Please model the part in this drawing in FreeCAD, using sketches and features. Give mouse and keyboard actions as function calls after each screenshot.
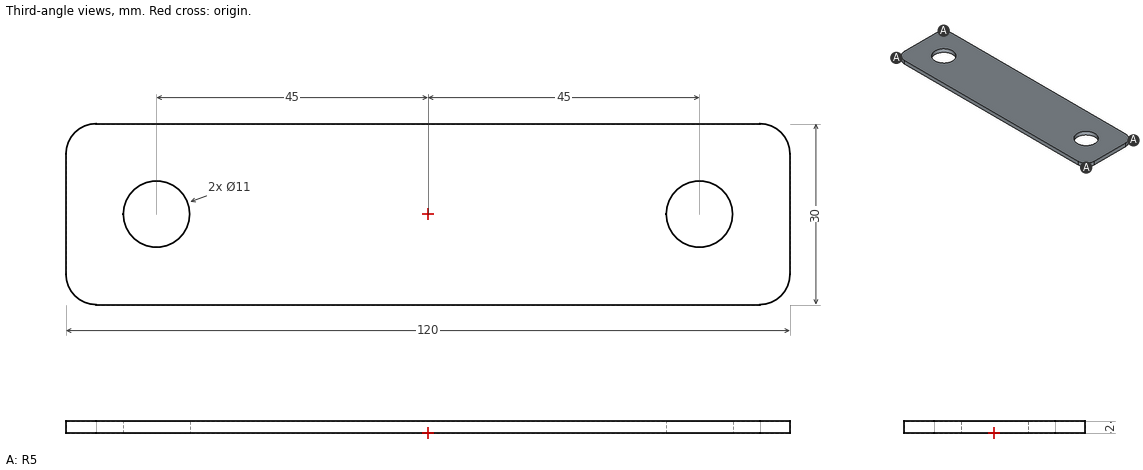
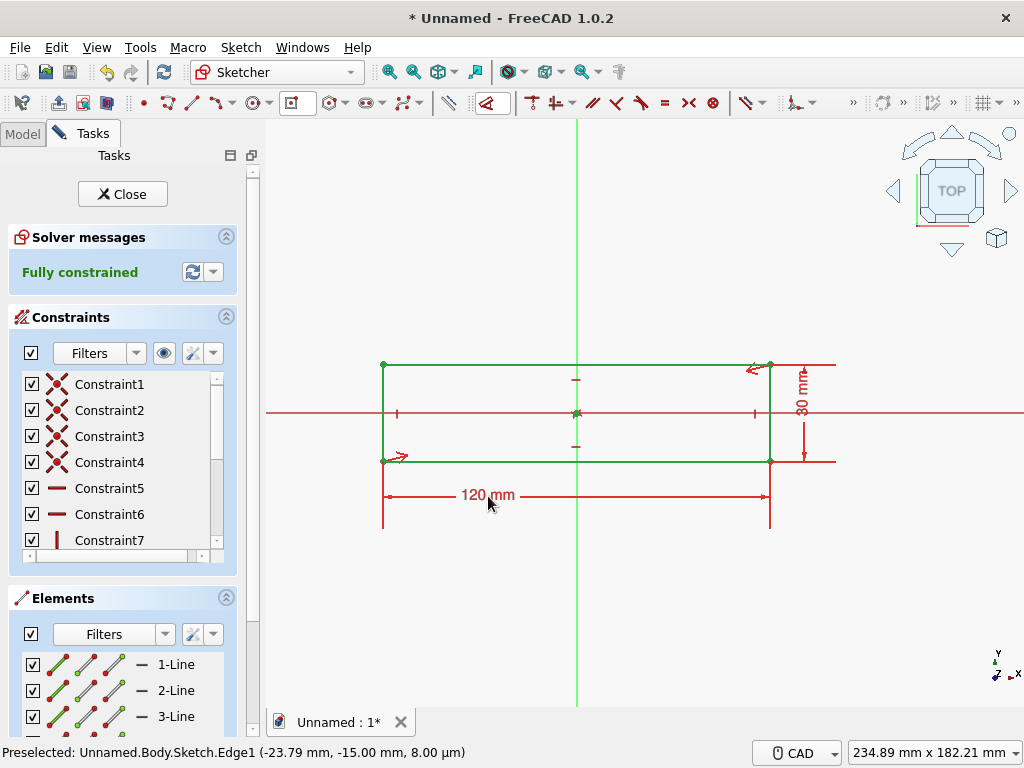
click(123, 194)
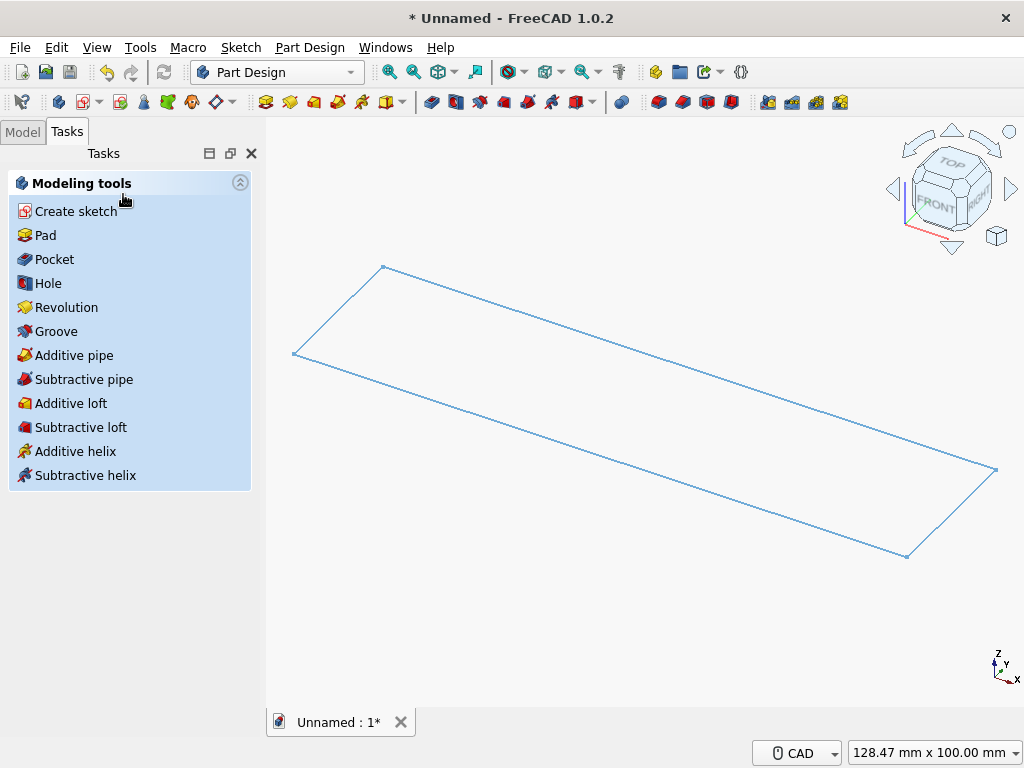
click(266, 102)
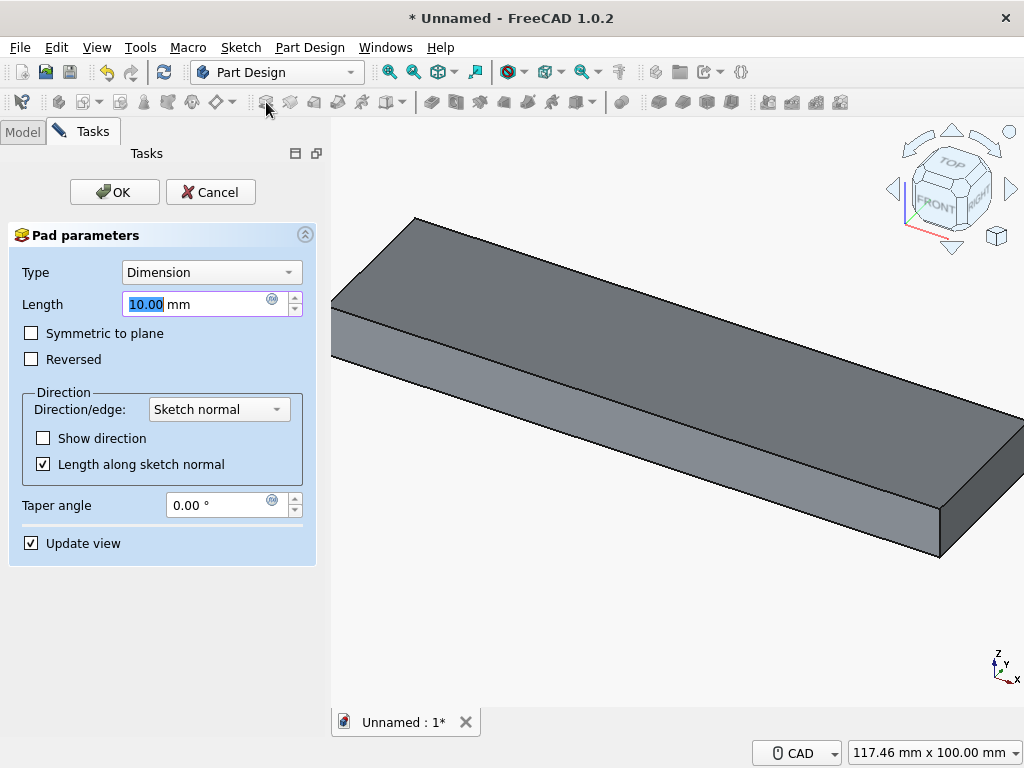
text(2)
key(Tab)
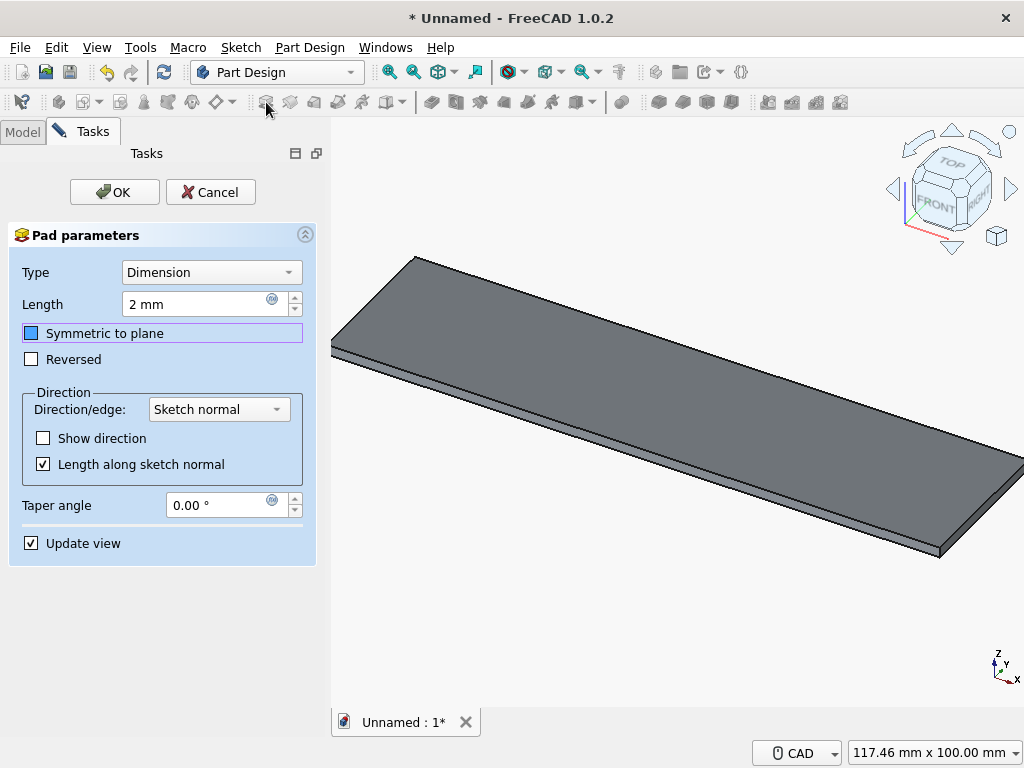
click(115, 192)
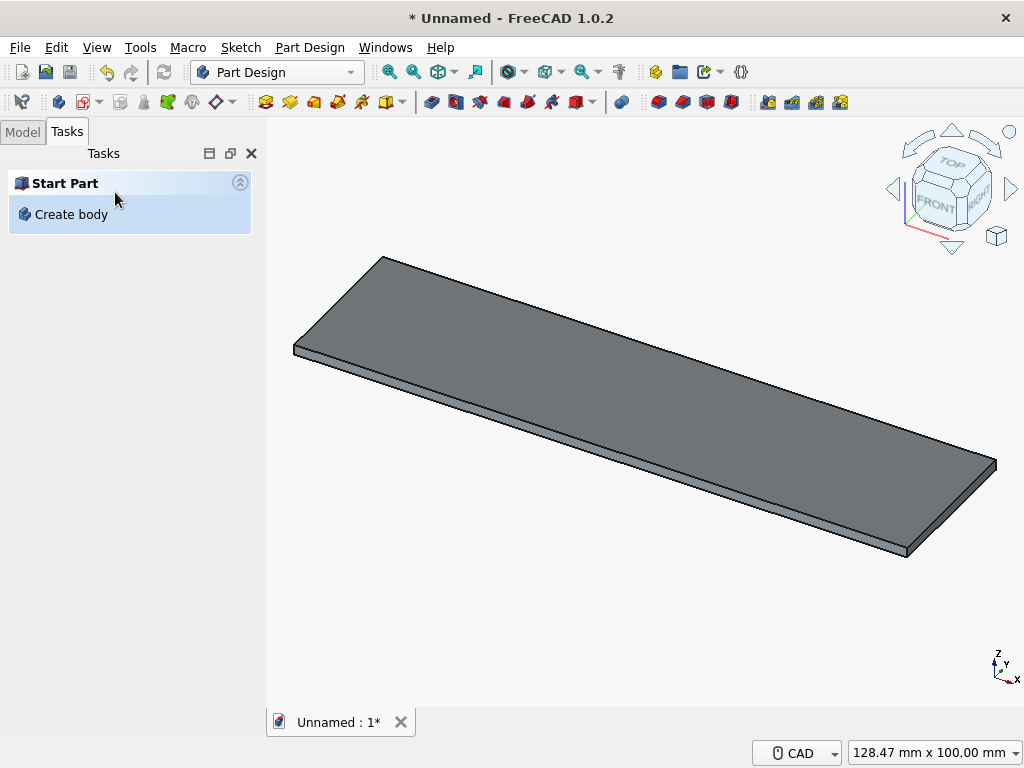
click(84, 102)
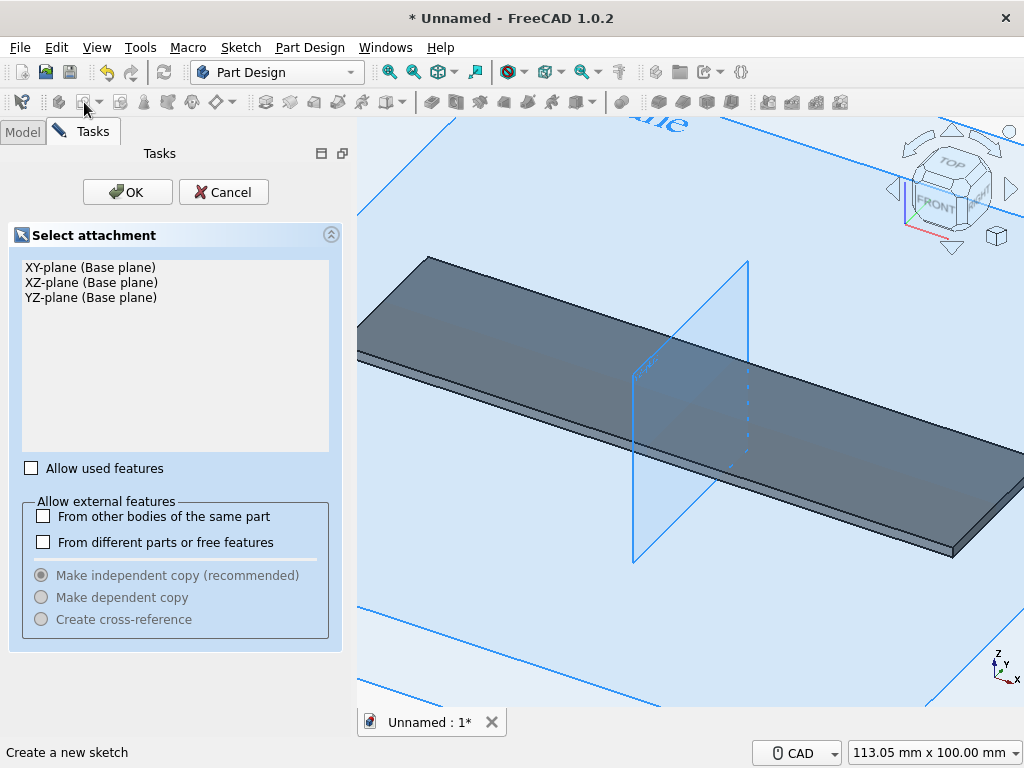
click(82, 268)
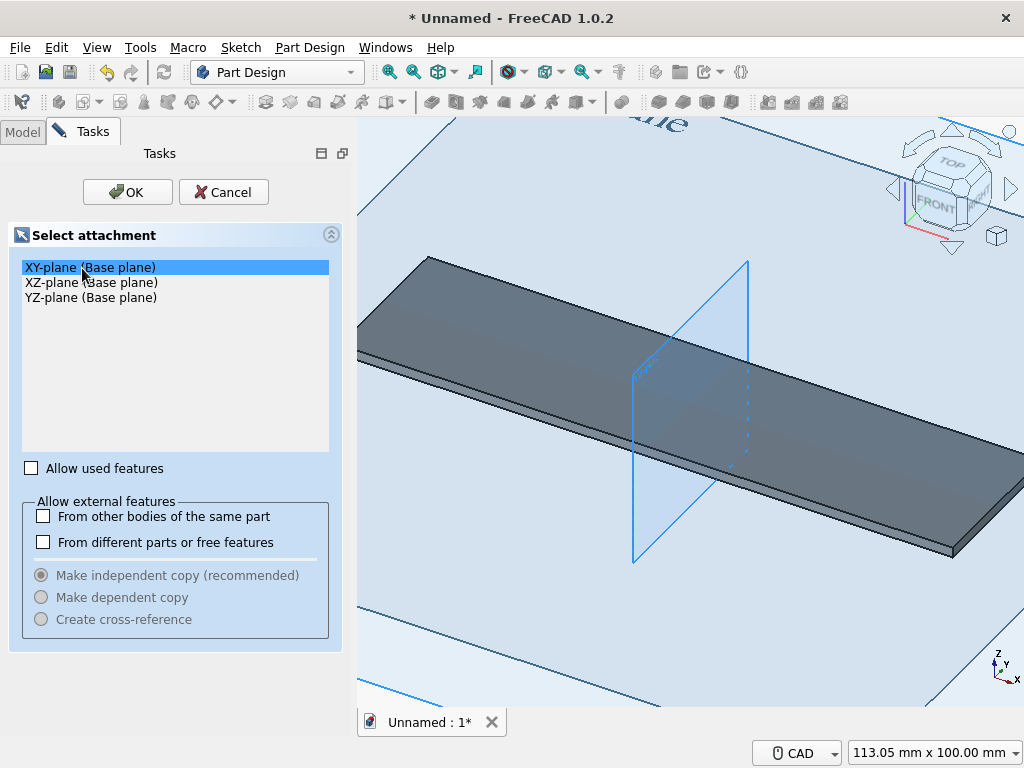
click(128, 192)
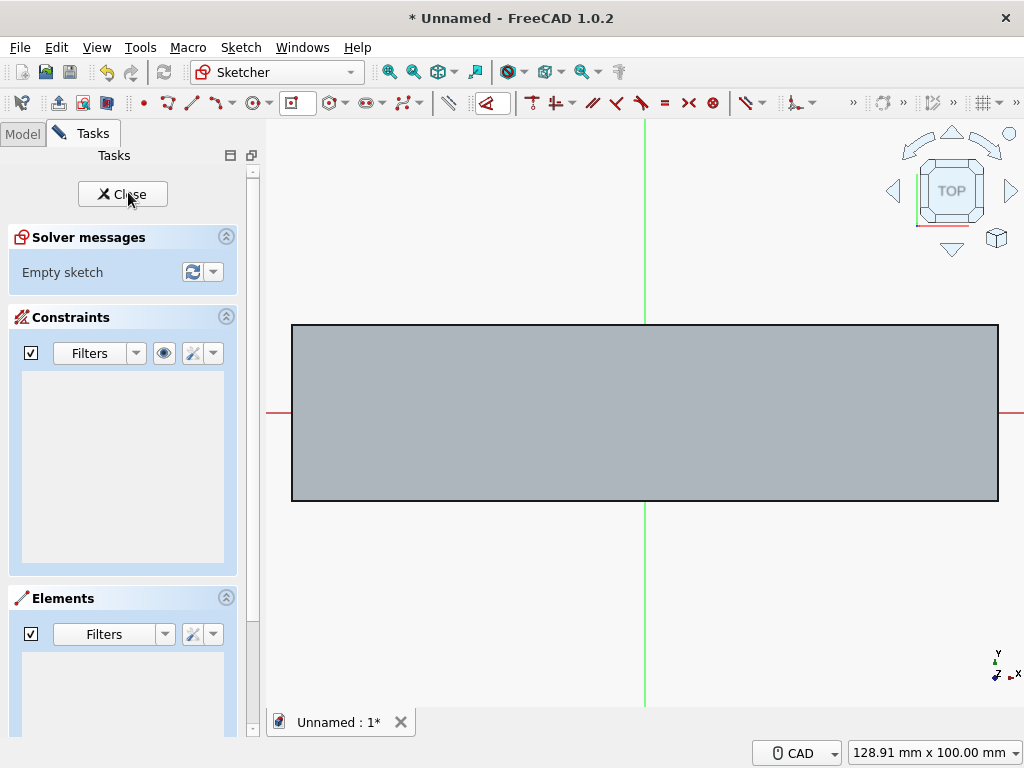
key(q)
key(s)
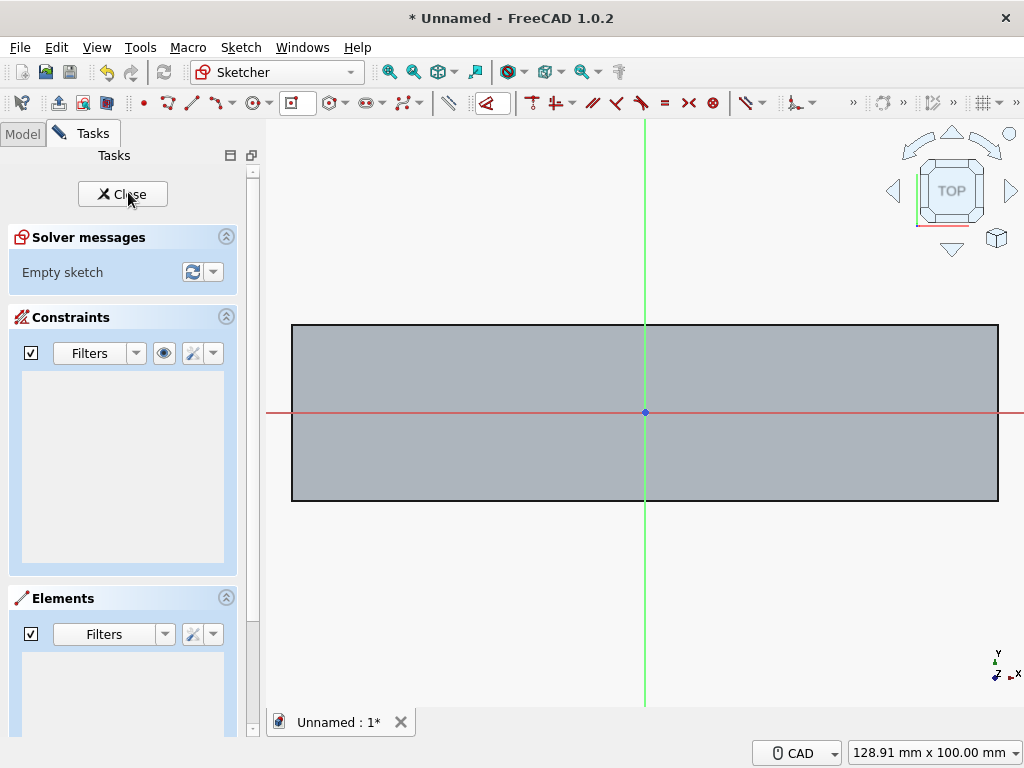
scroll(437, 413, down, 2)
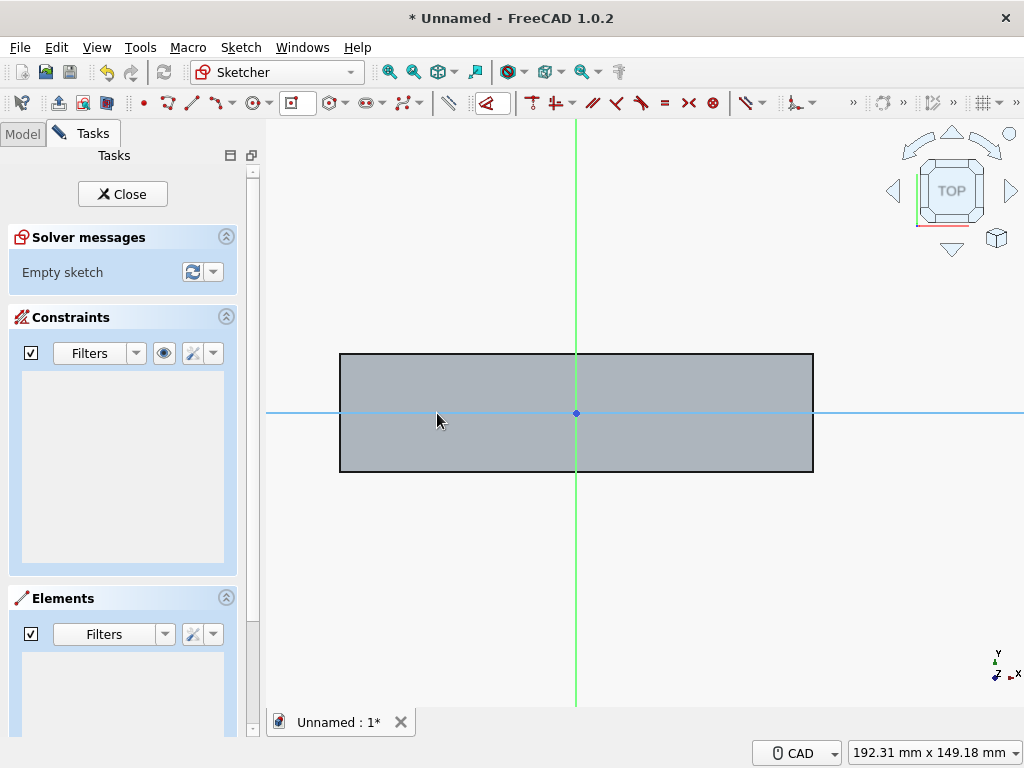
click(254, 104)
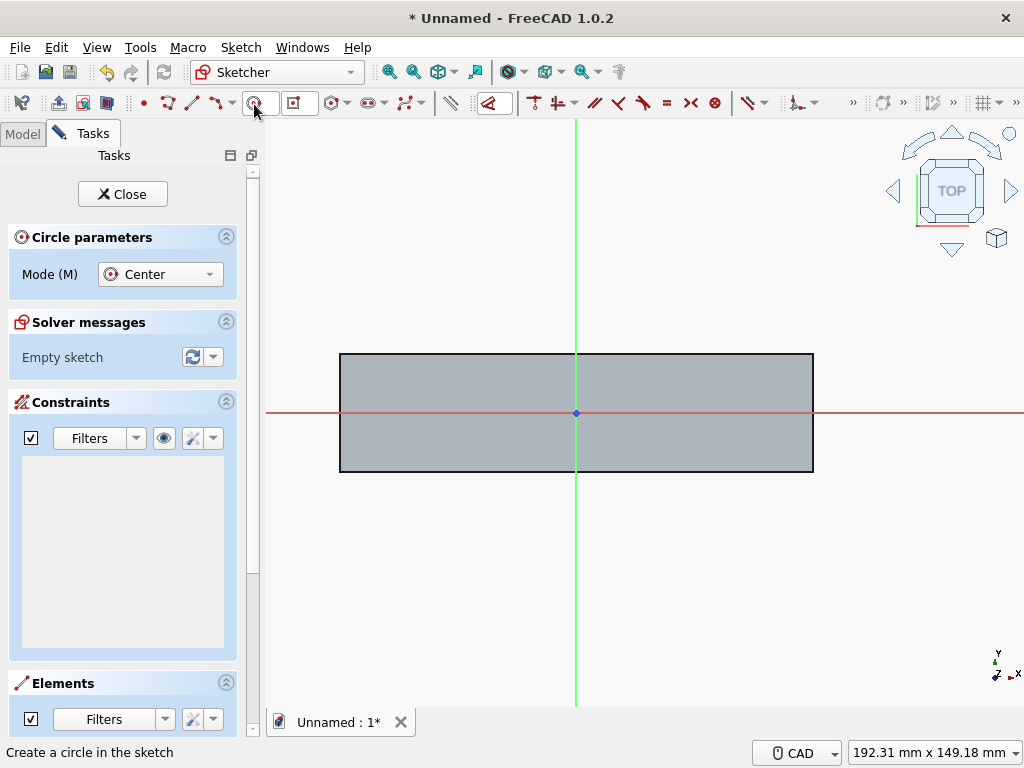
click(399, 413)
click(414, 398)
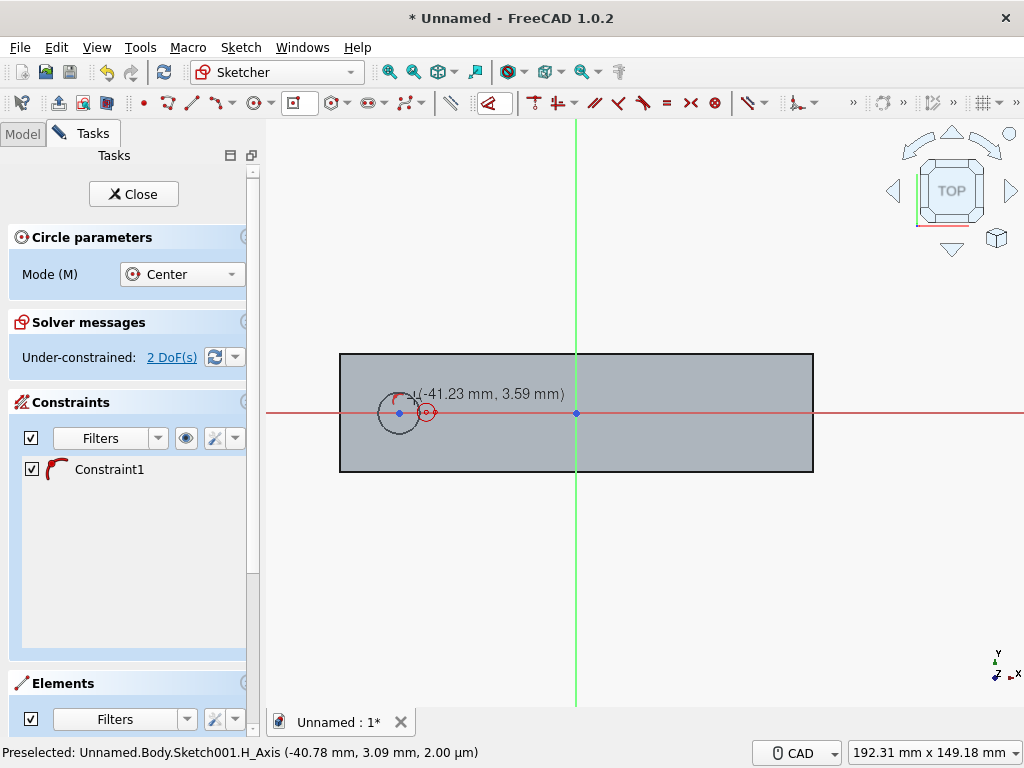
click(754, 413)
click(769, 398)
key(Escape)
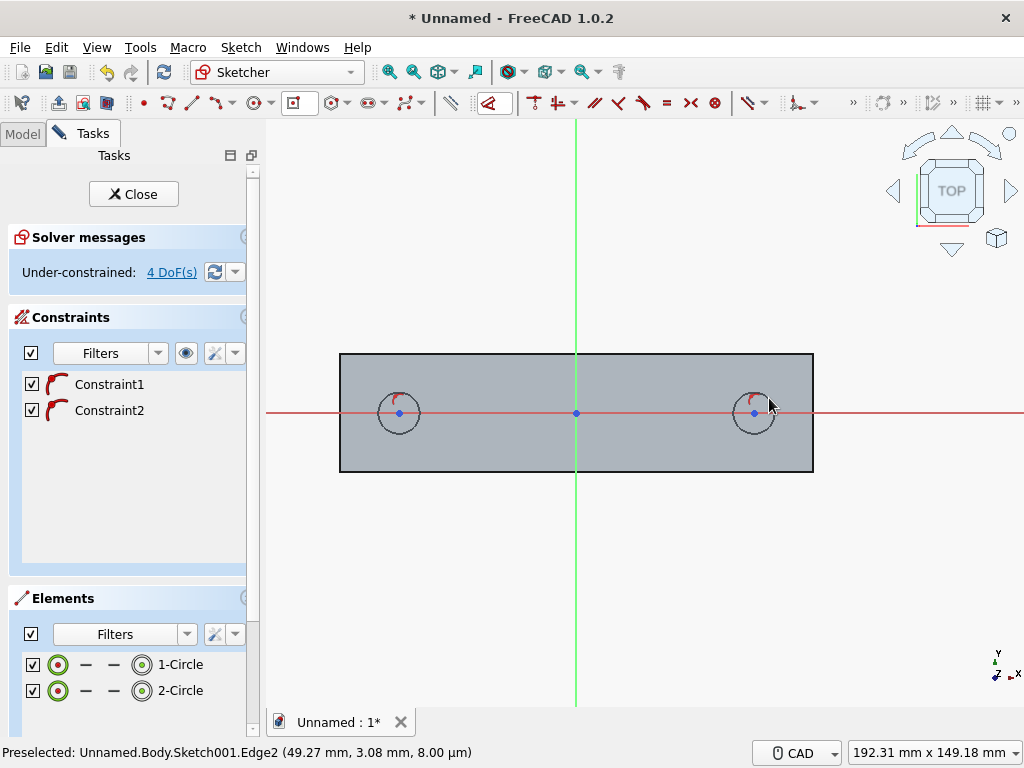
click(414, 399)